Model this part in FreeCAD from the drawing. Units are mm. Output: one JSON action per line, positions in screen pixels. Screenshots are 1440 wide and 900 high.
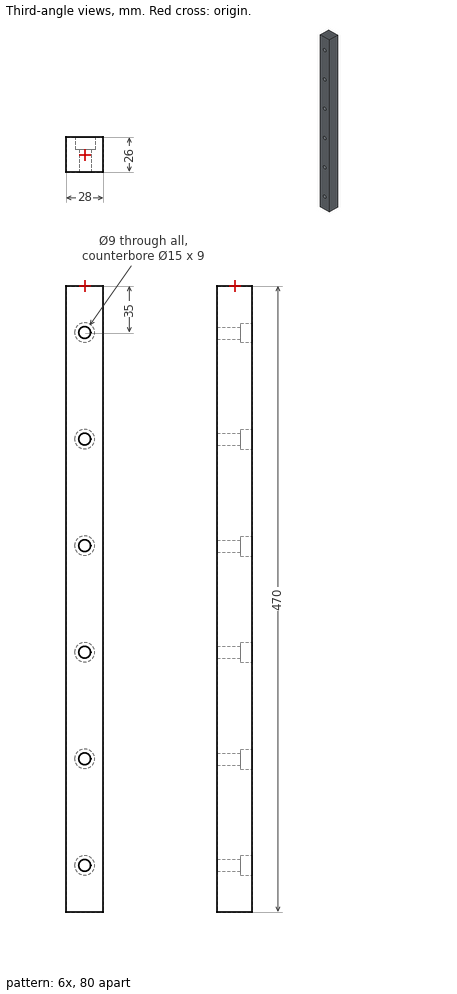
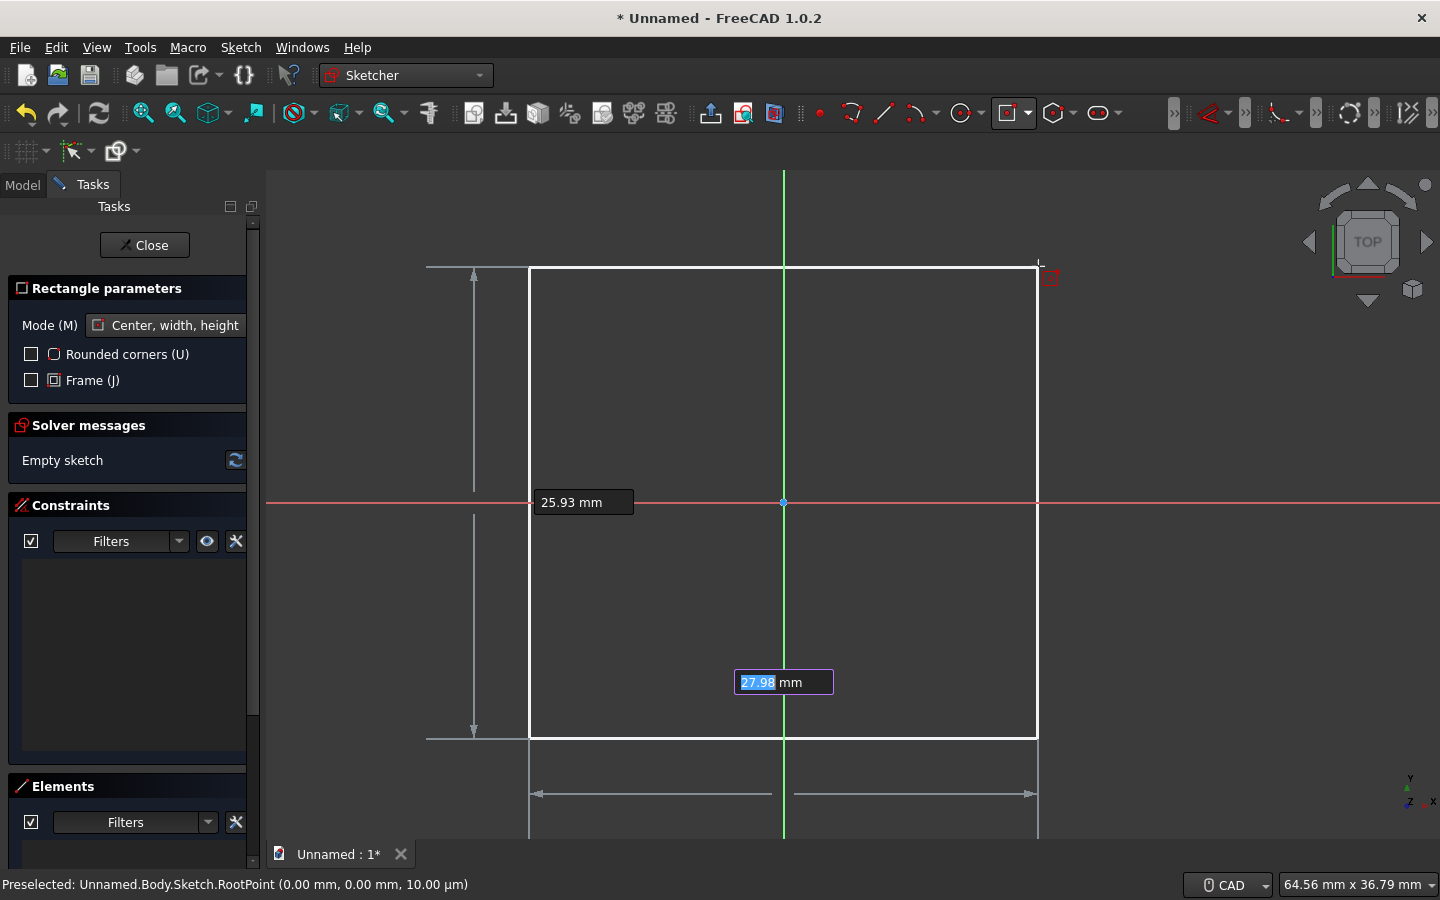
{"action": "type", "text": "28"}
{"action": "key", "text": "Tab"}
{"action": "type", "text": "26"}
{"action": "key", "text": "Return"}
{"action": "key", "text": "Escape"}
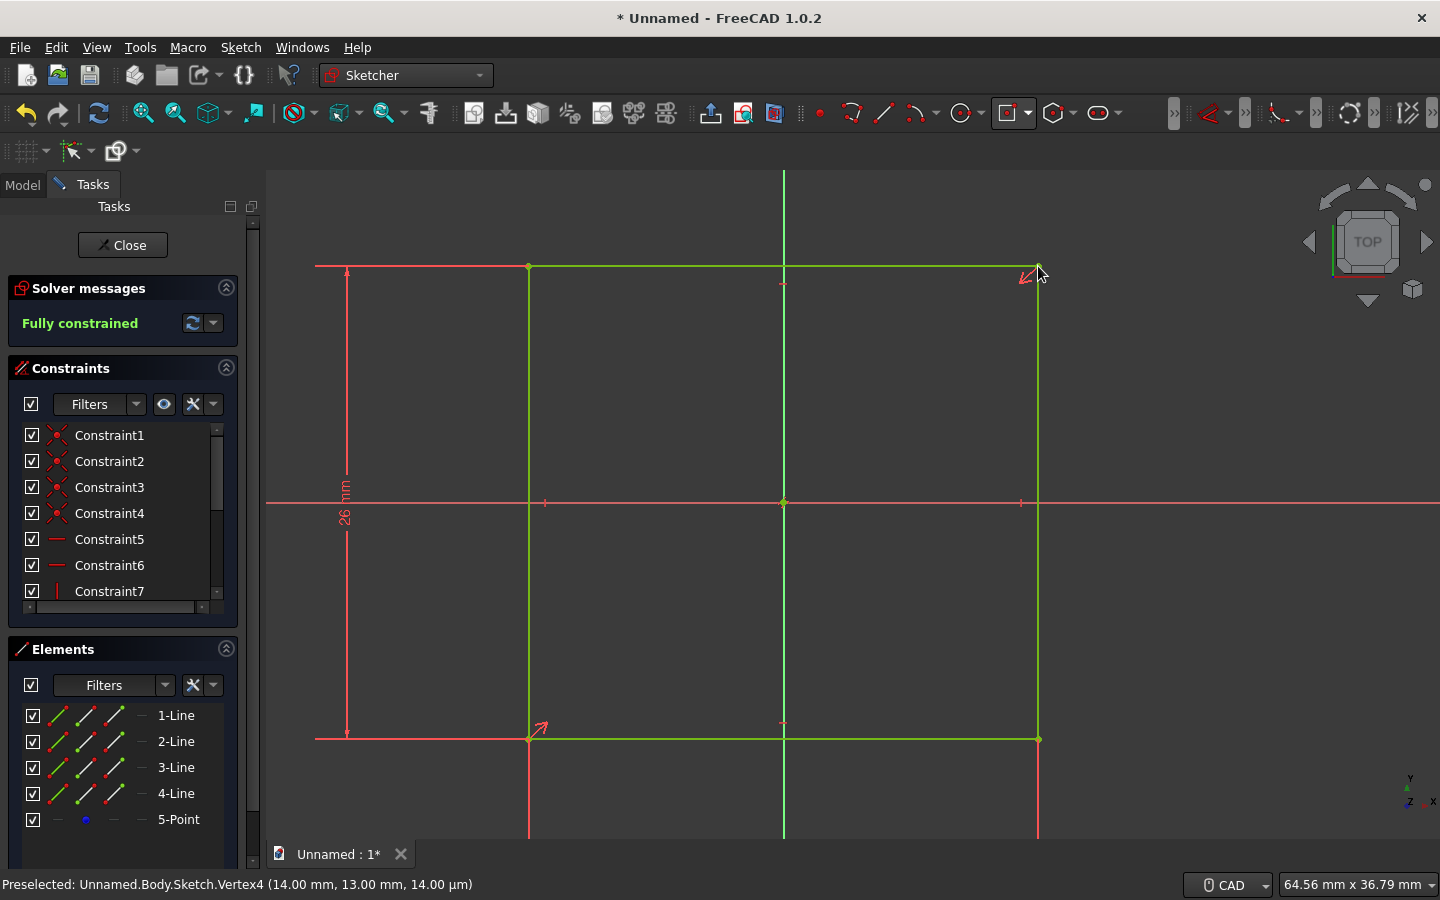
{"action": "left_click", "coordinate": [123, 245]}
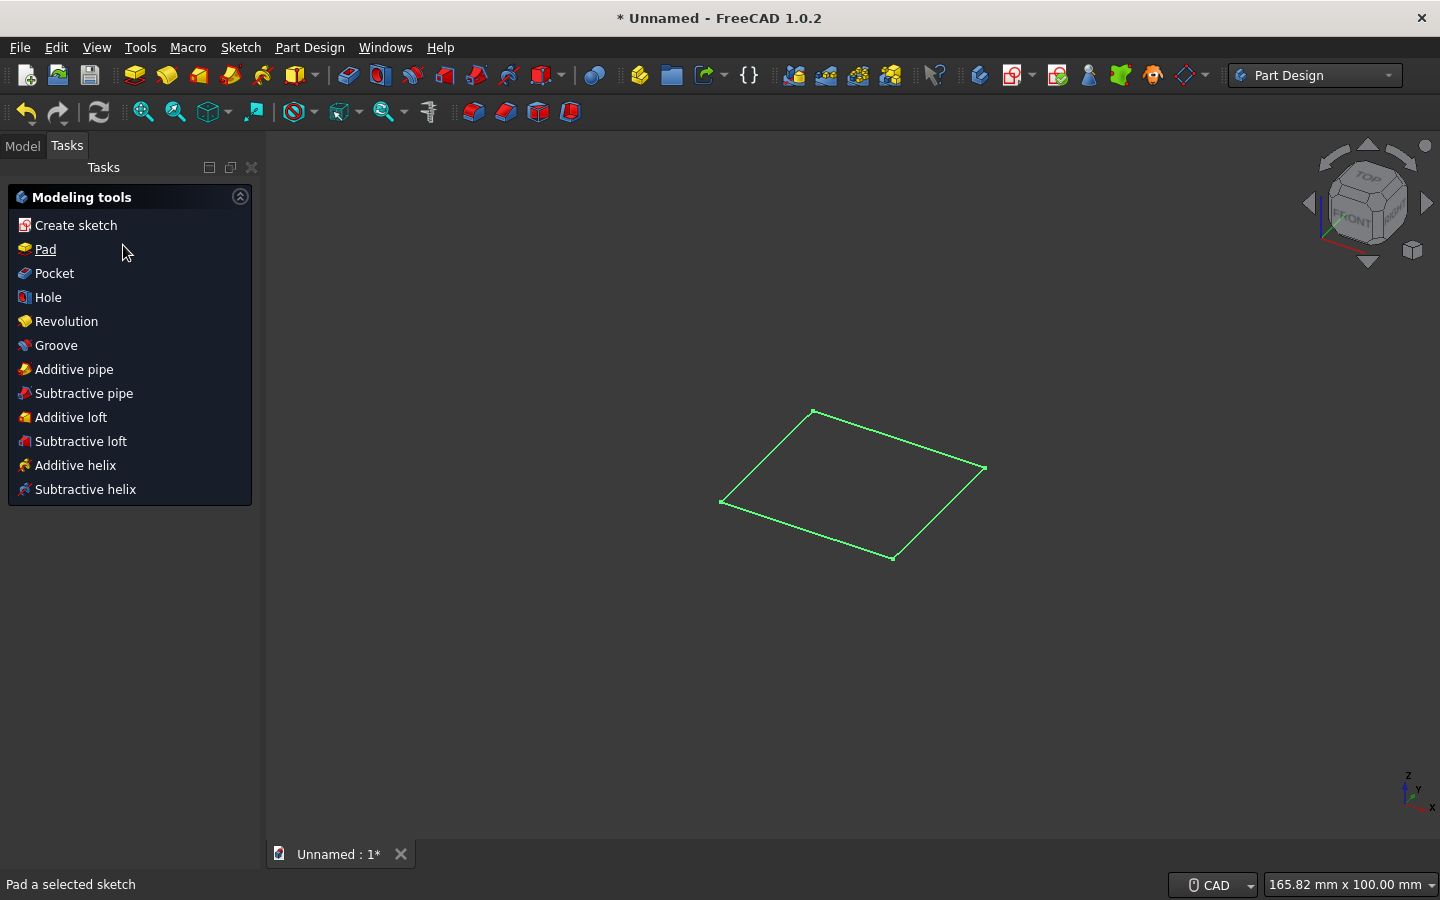
{"action": "left_click", "coordinate": [136, 76]}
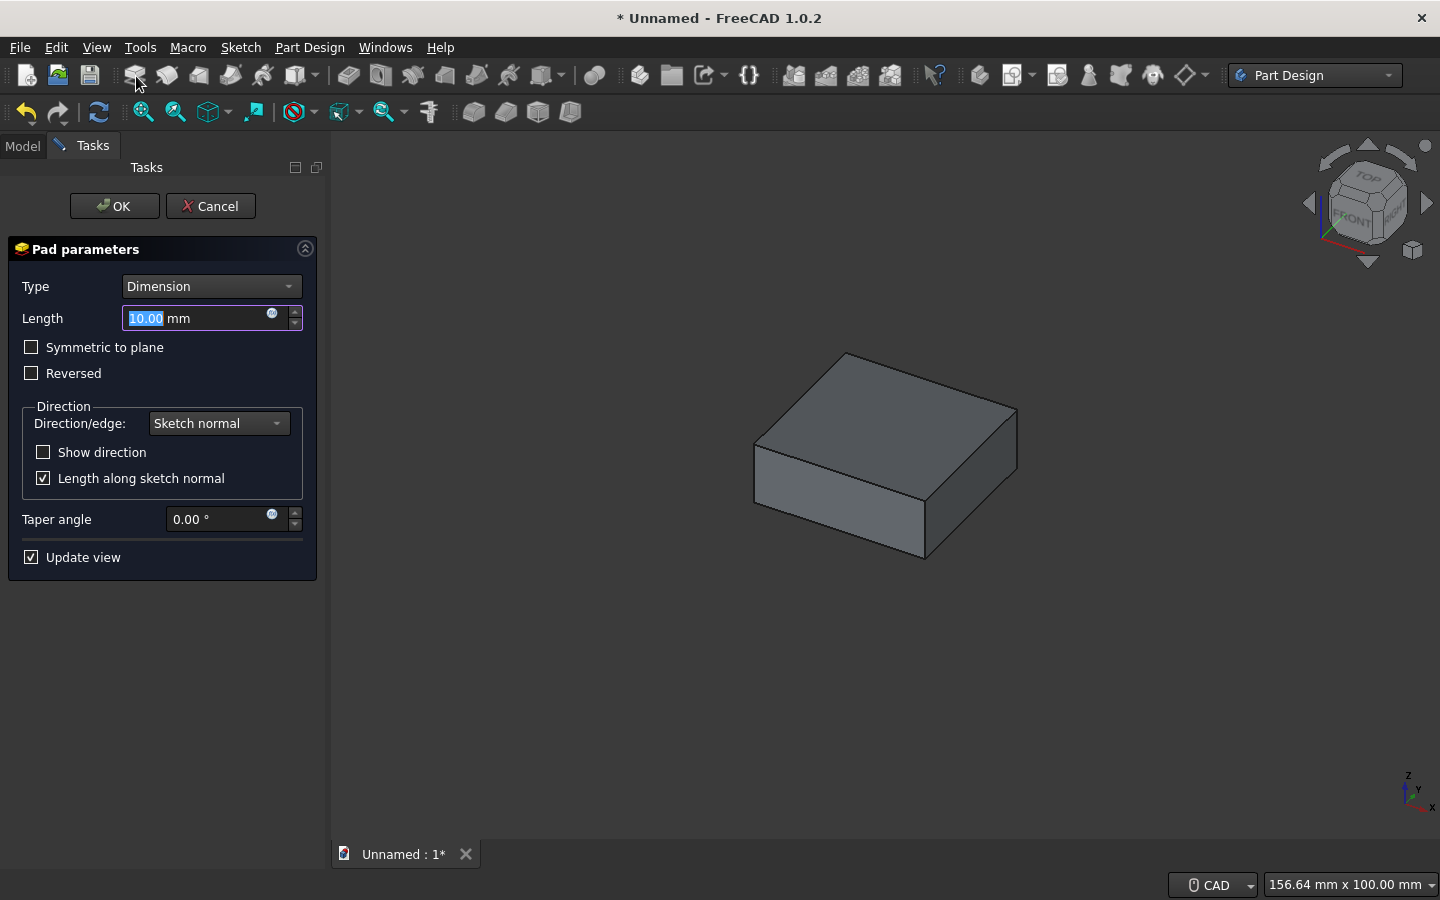
{"action": "type", "text": "470"}
{"action": "key", "text": "Tab"}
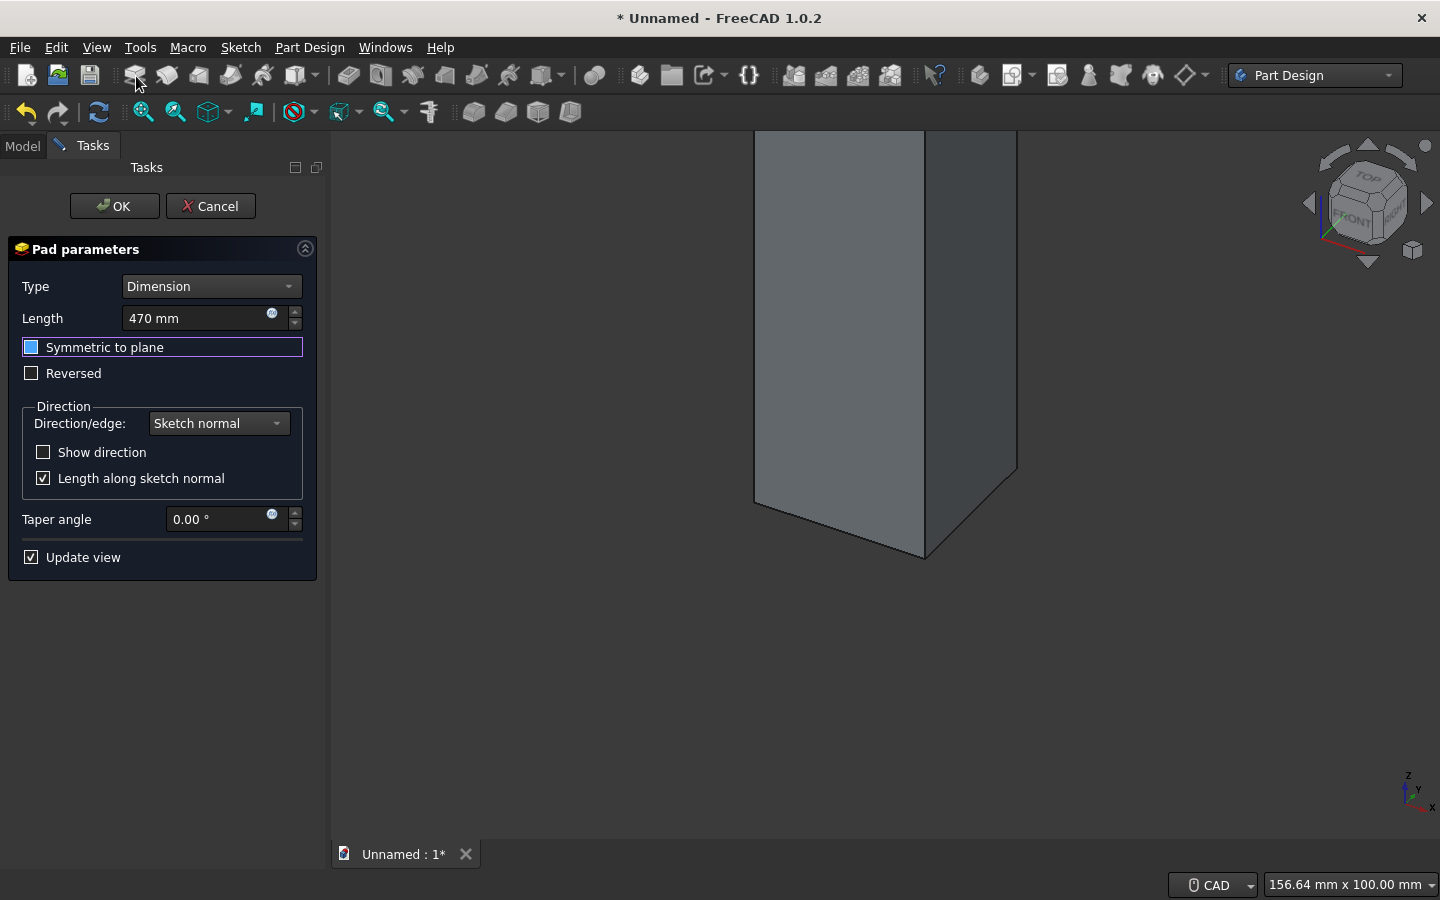
{"action": "left_click", "coordinate": [30, 373]}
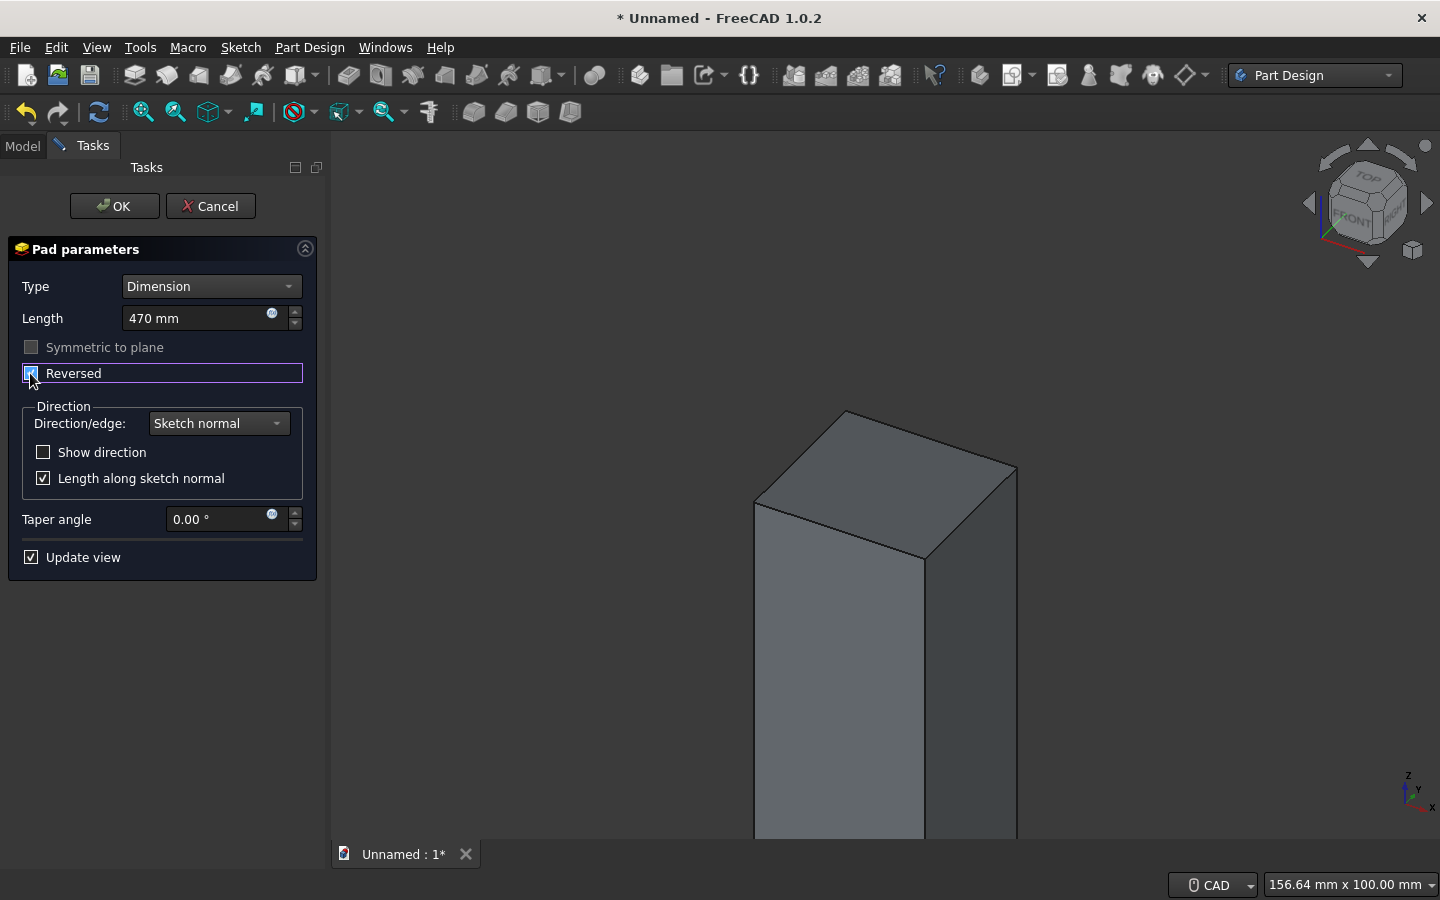
{"action": "left_click", "coordinate": [115, 206]}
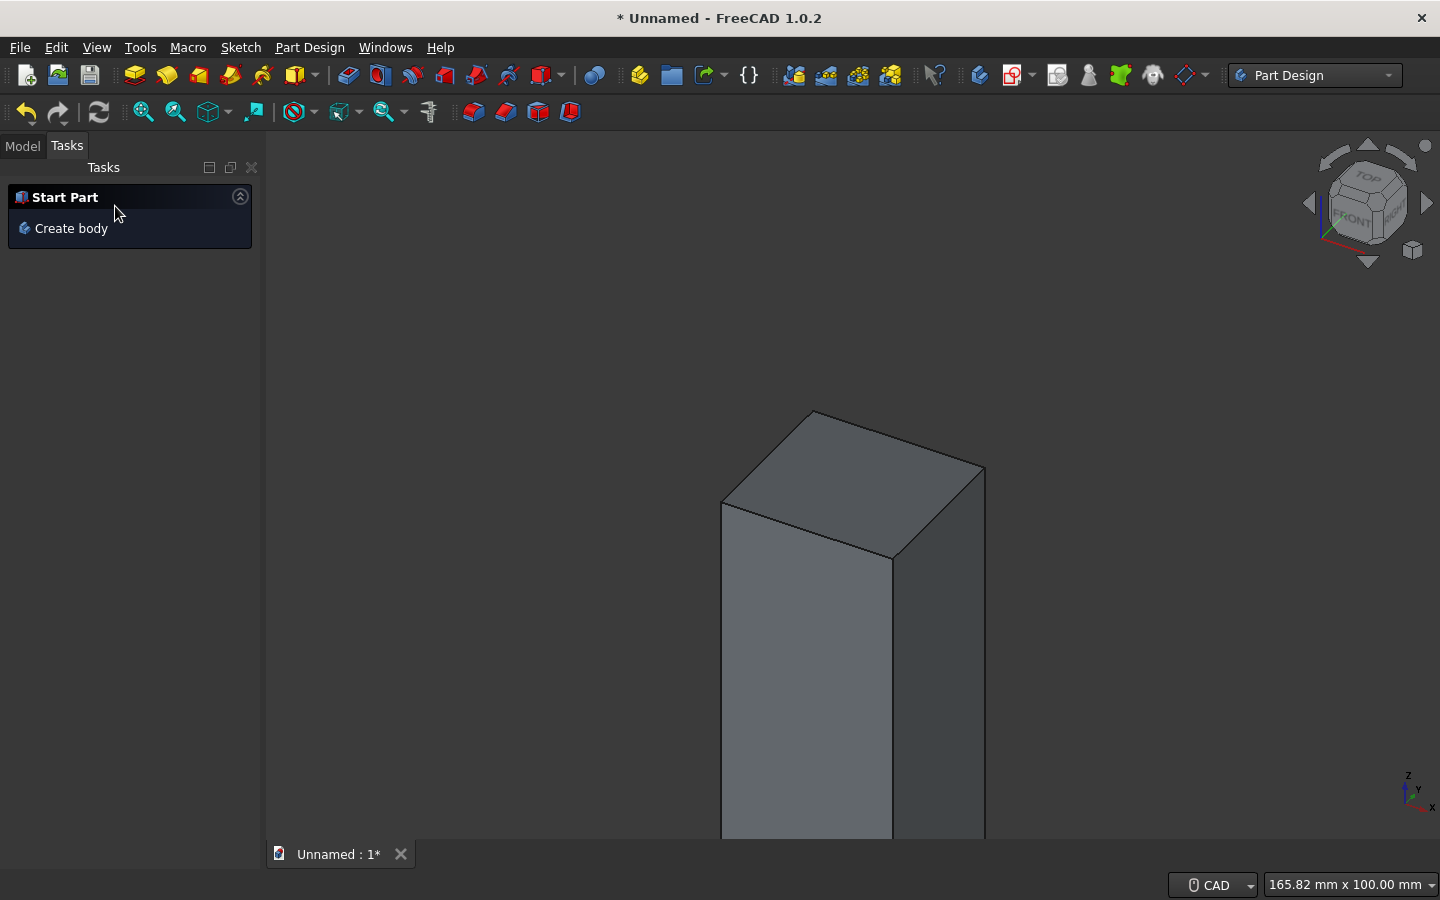
{"action": "left_click", "coordinate": [144, 112]}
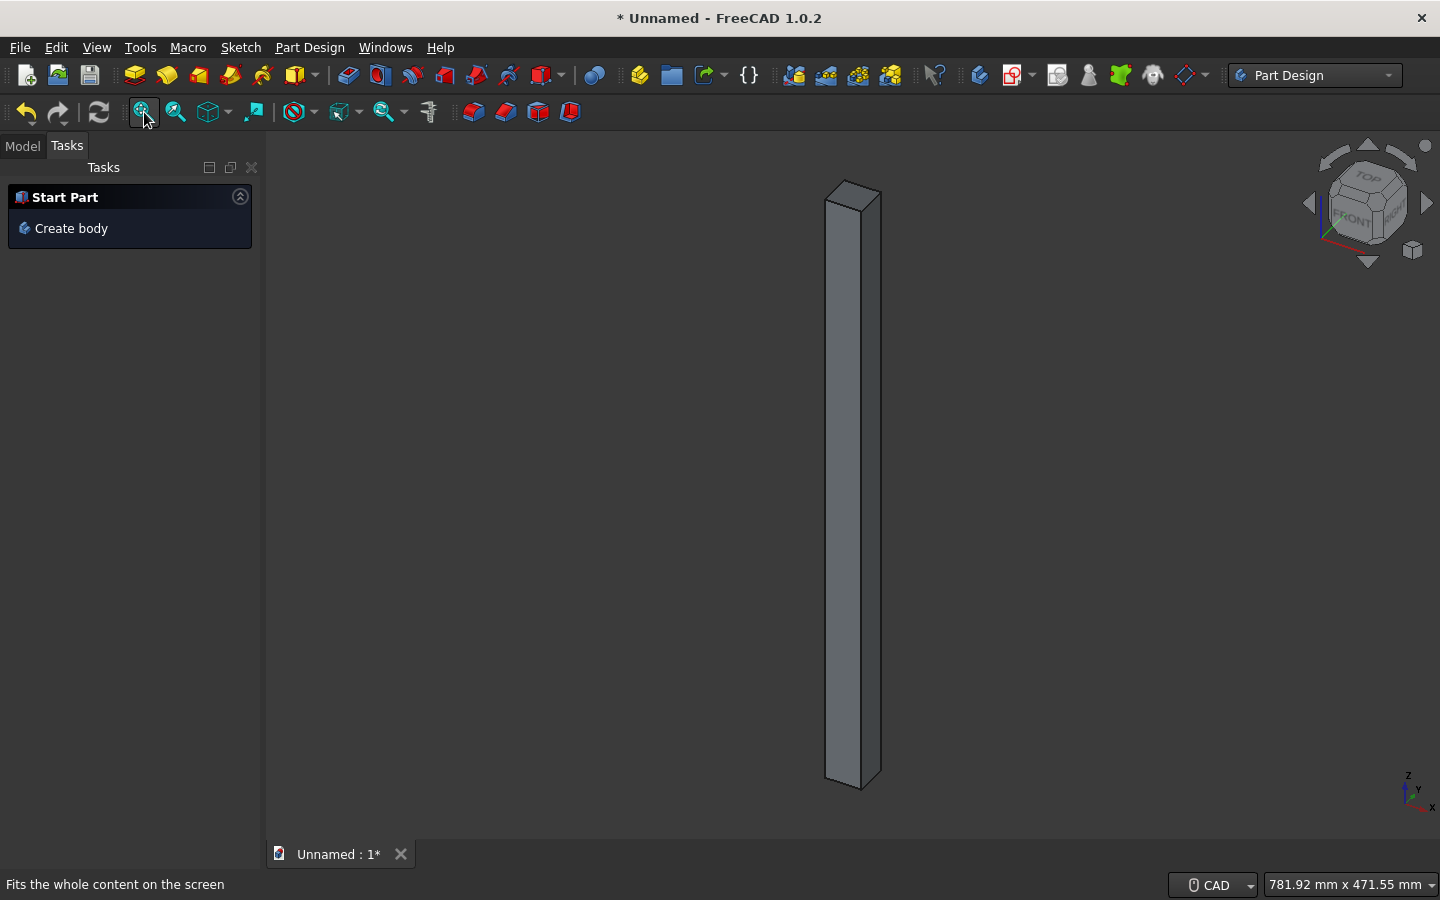
{"action": "key", "text": "4"}